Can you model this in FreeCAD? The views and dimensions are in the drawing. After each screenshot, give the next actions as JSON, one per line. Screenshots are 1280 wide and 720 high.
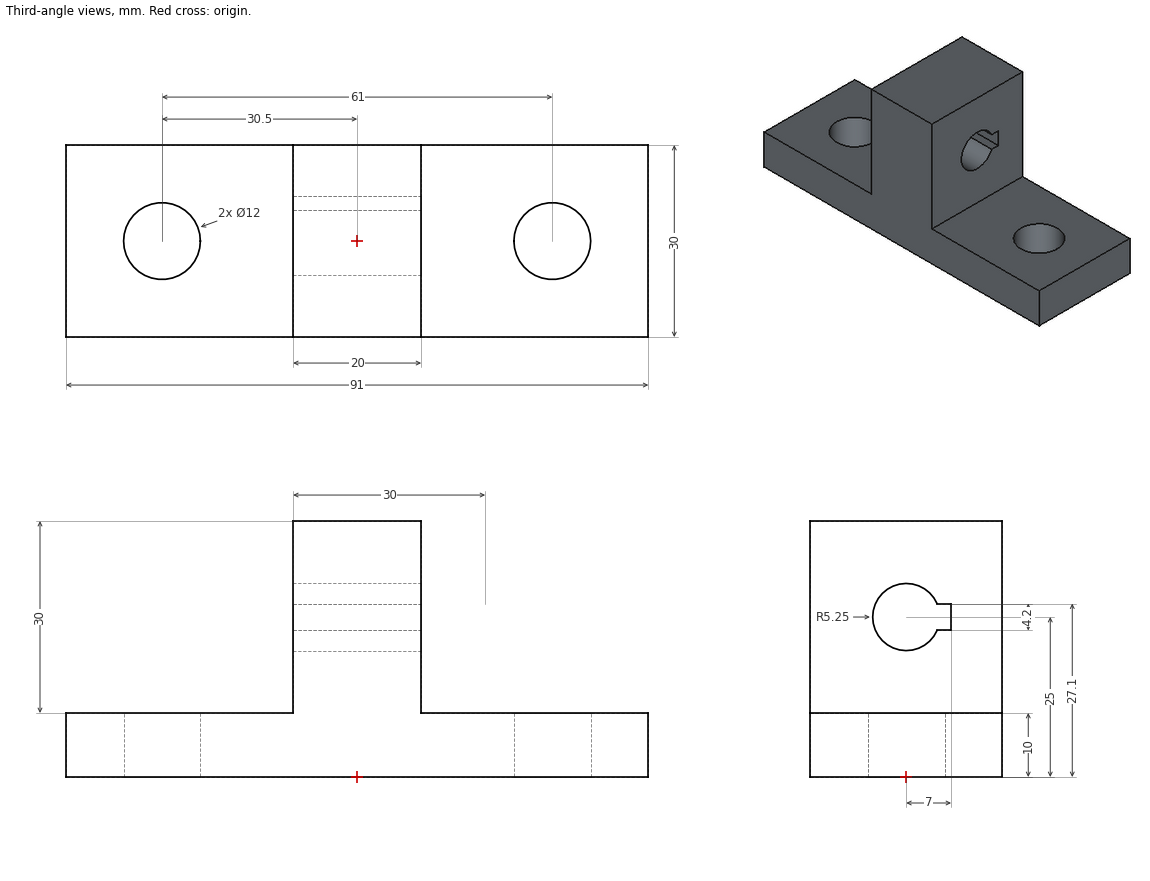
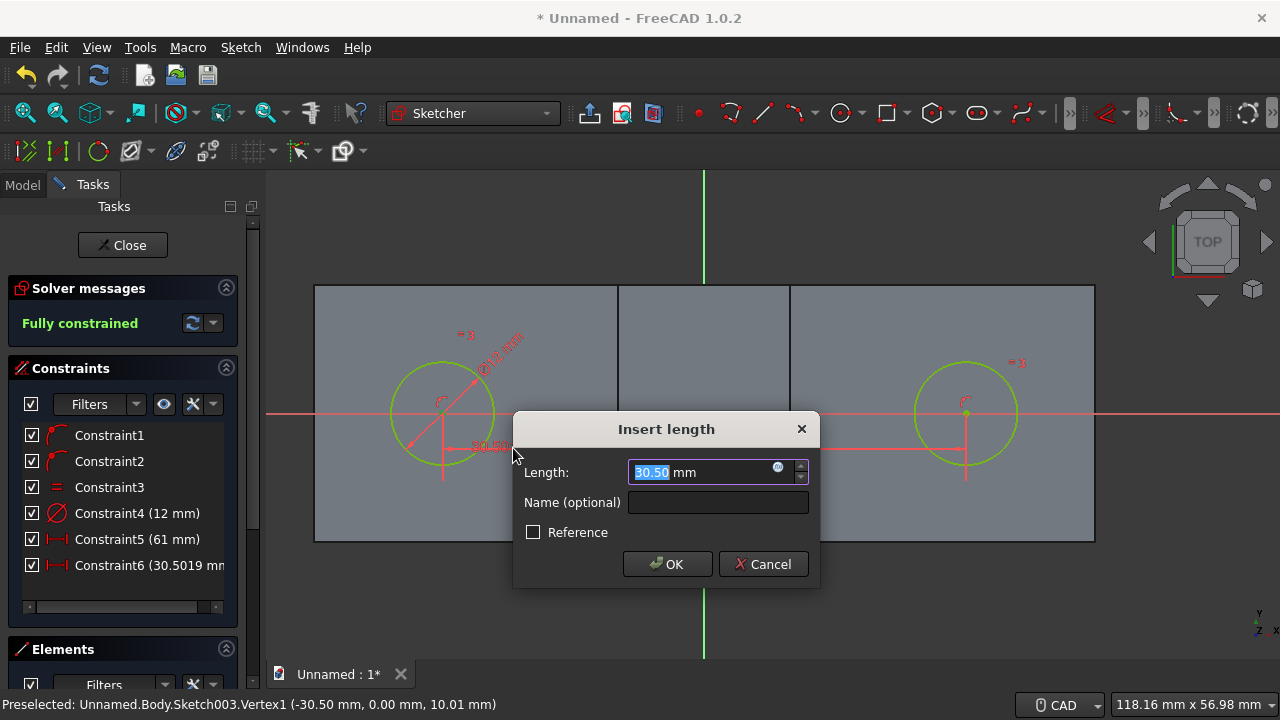
{"action": "type", "text": "30.5"}
{"action": "key", "text": "Return"}
{"action": "key", "text": "Escape"}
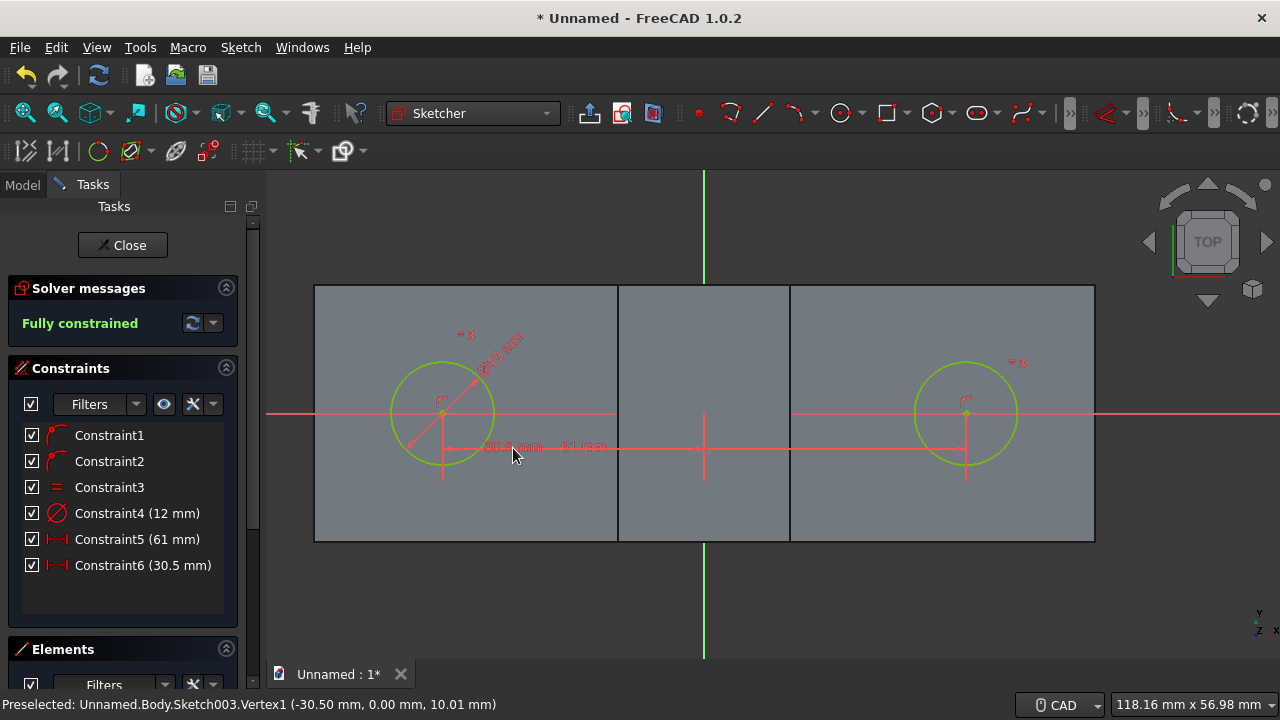
{"action": "left_click", "coordinate": [123, 245]}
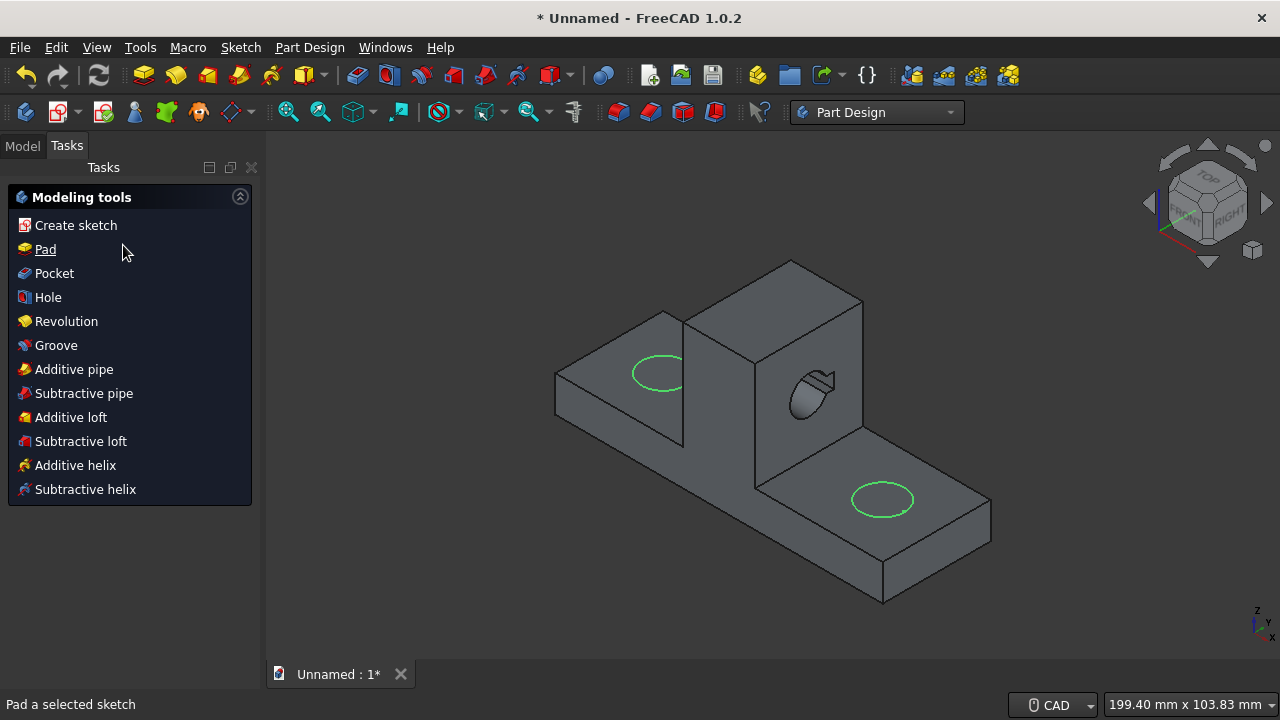
{"action": "left_click", "coordinate": [358, 76]}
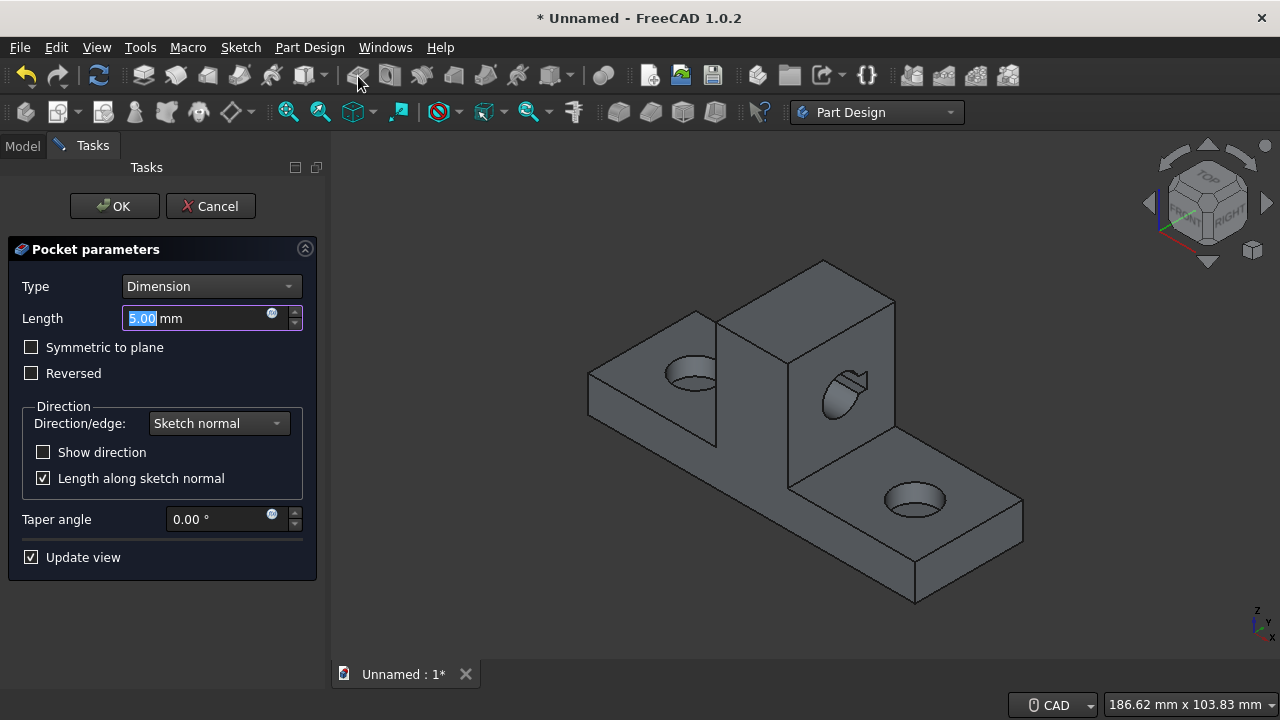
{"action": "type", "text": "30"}
{"action": "key", "text": "Tab"}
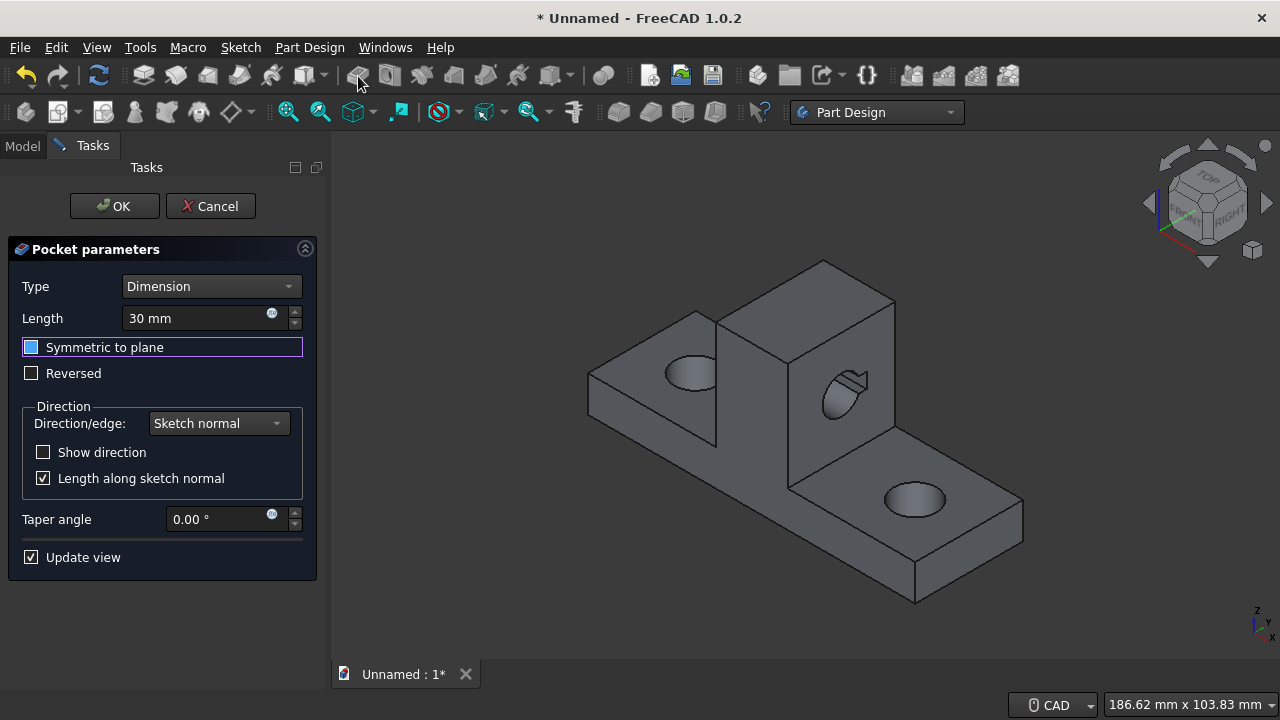
{"action": "left_click", "coordinate": [115, 206]}